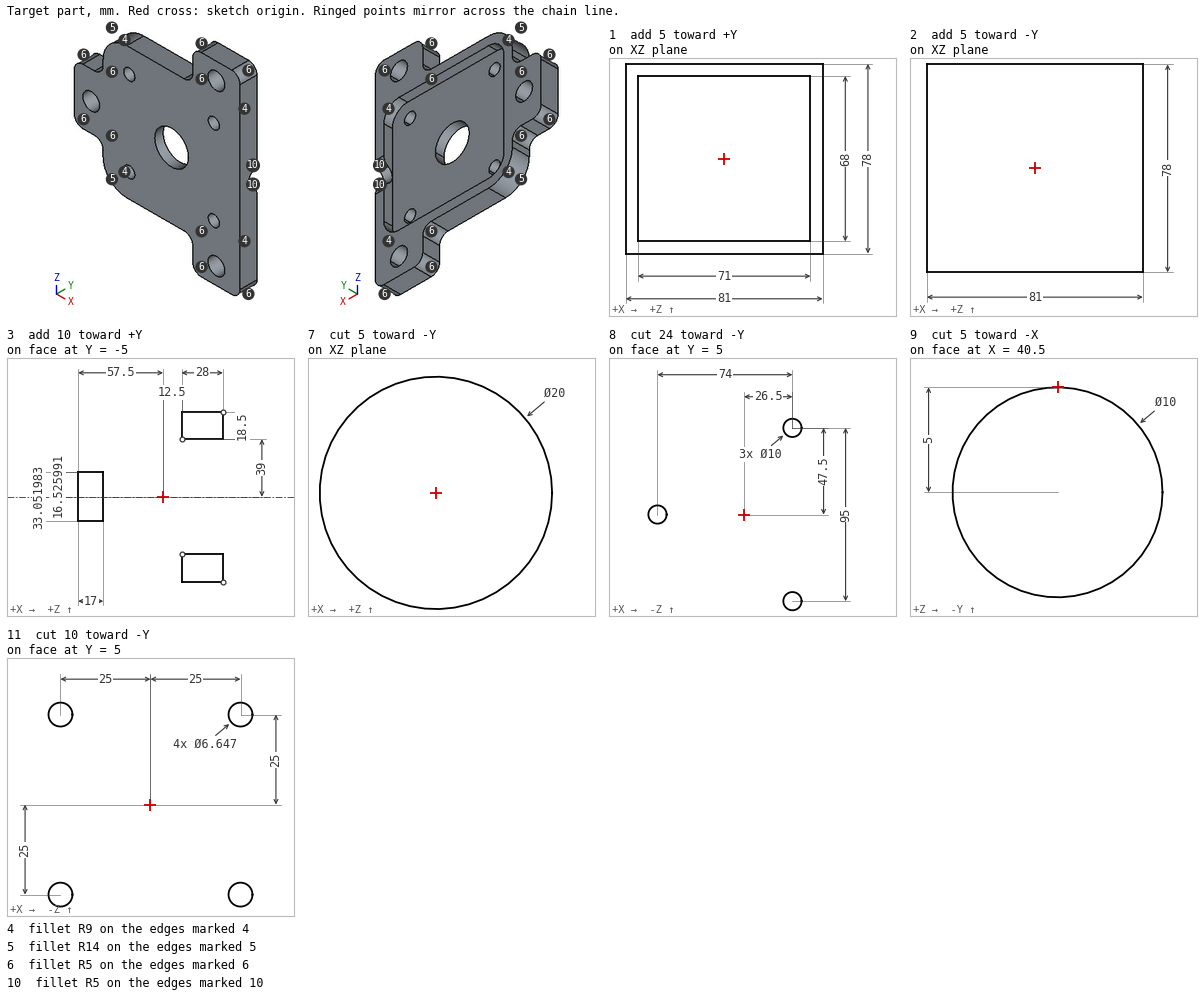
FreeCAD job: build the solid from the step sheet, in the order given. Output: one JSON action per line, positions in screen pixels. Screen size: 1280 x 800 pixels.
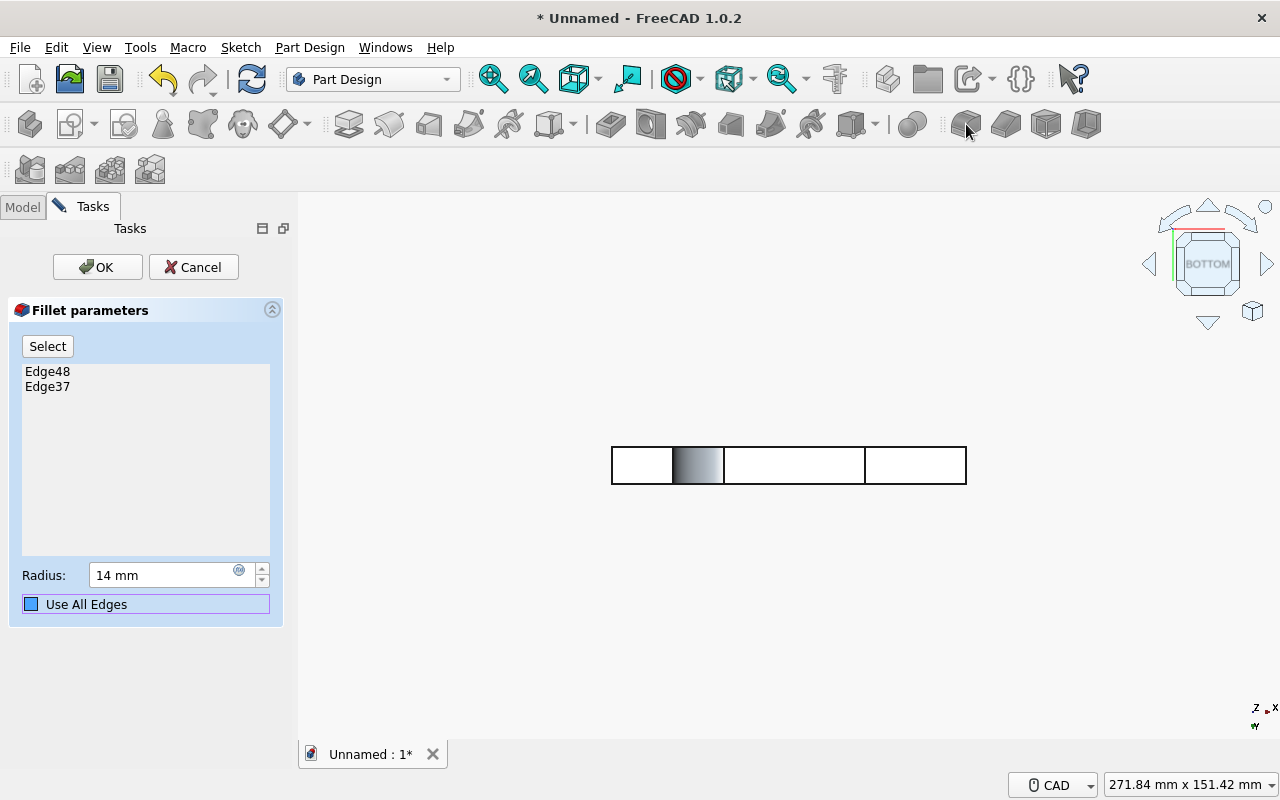
{"action": "left_click", "coordinate": [98, 267]}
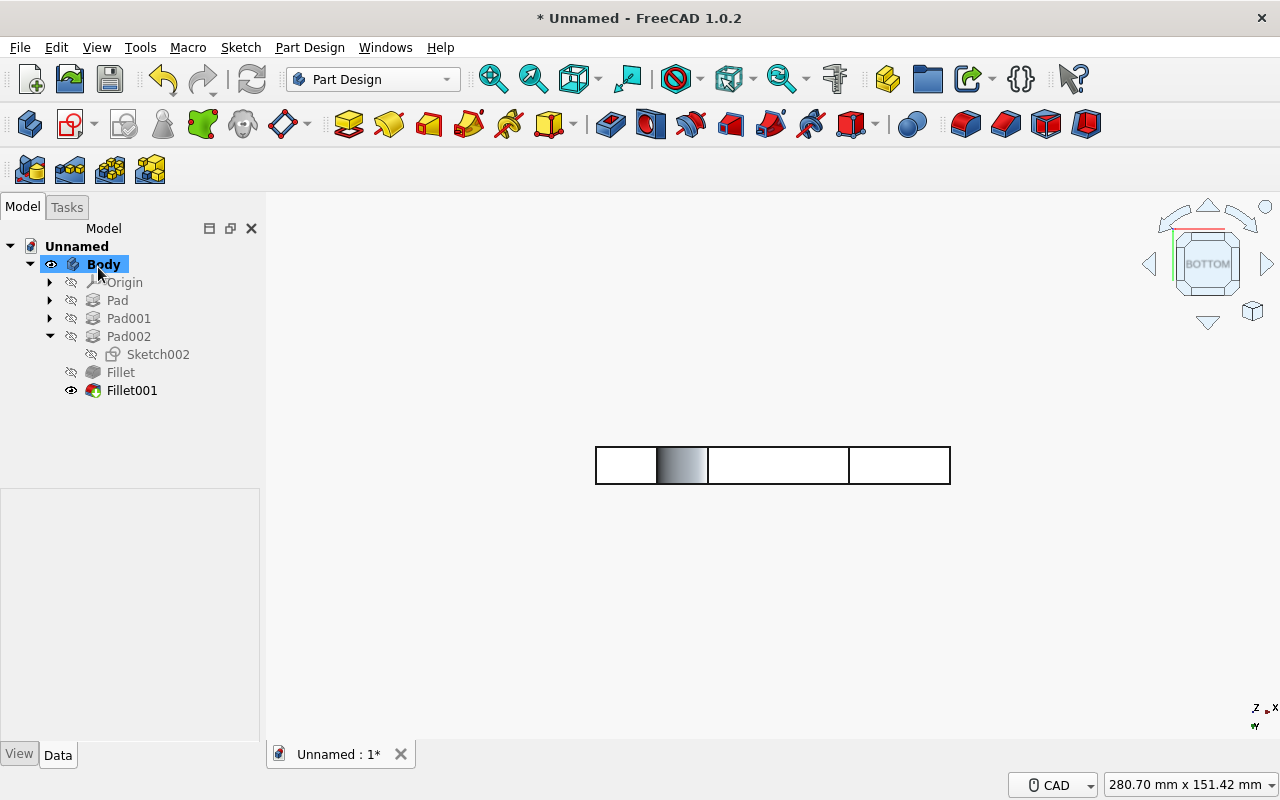
{"action": "left_click", "coordinate": [494, 80]}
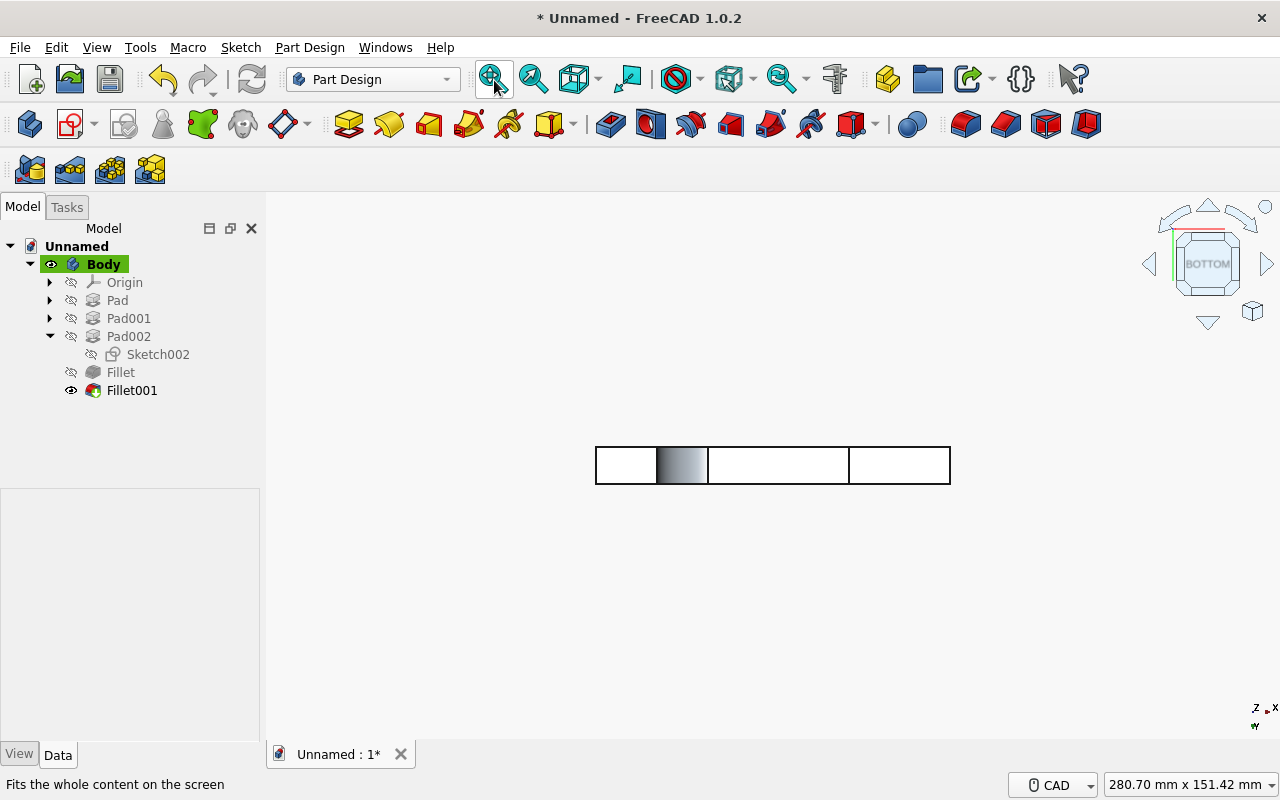
{"action": "left_click", "coordinate": [596, 464]}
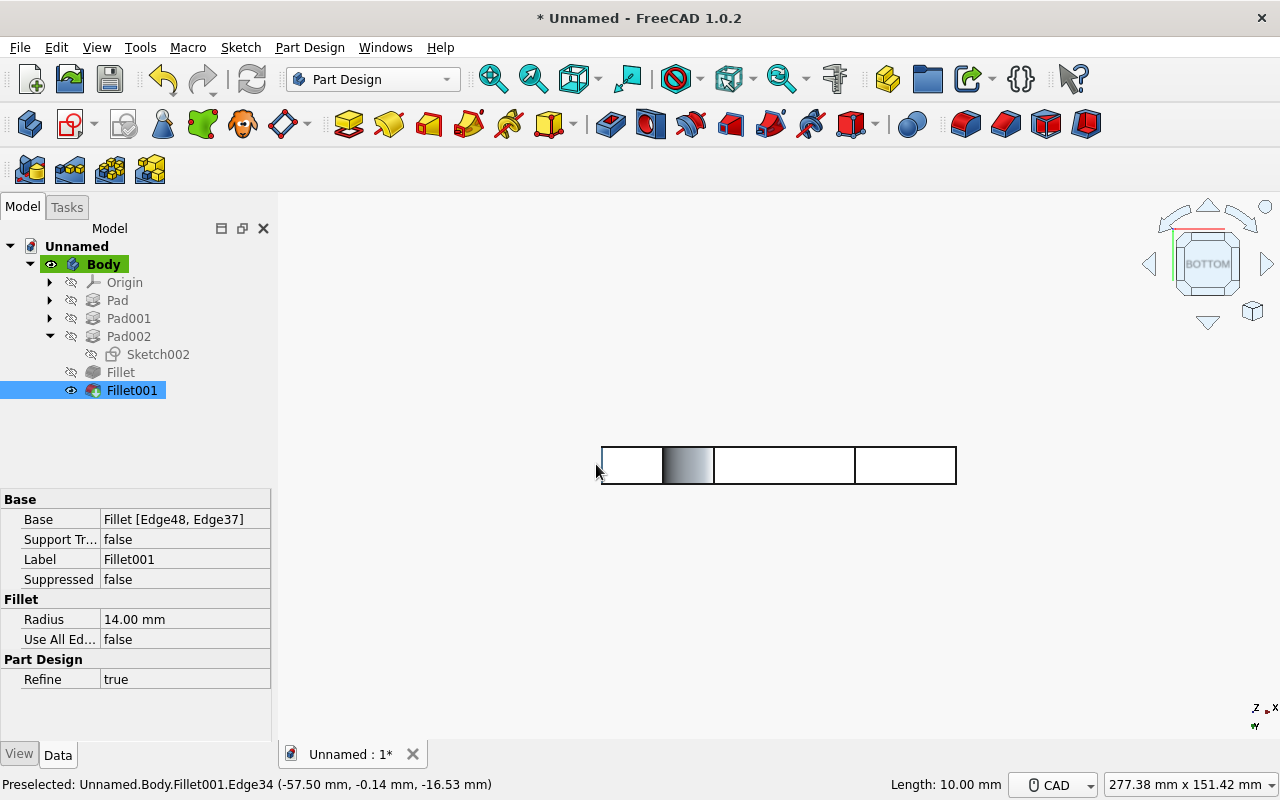
{"action": "left_click", "coordinate": [956, 464], "text": "ctrl"}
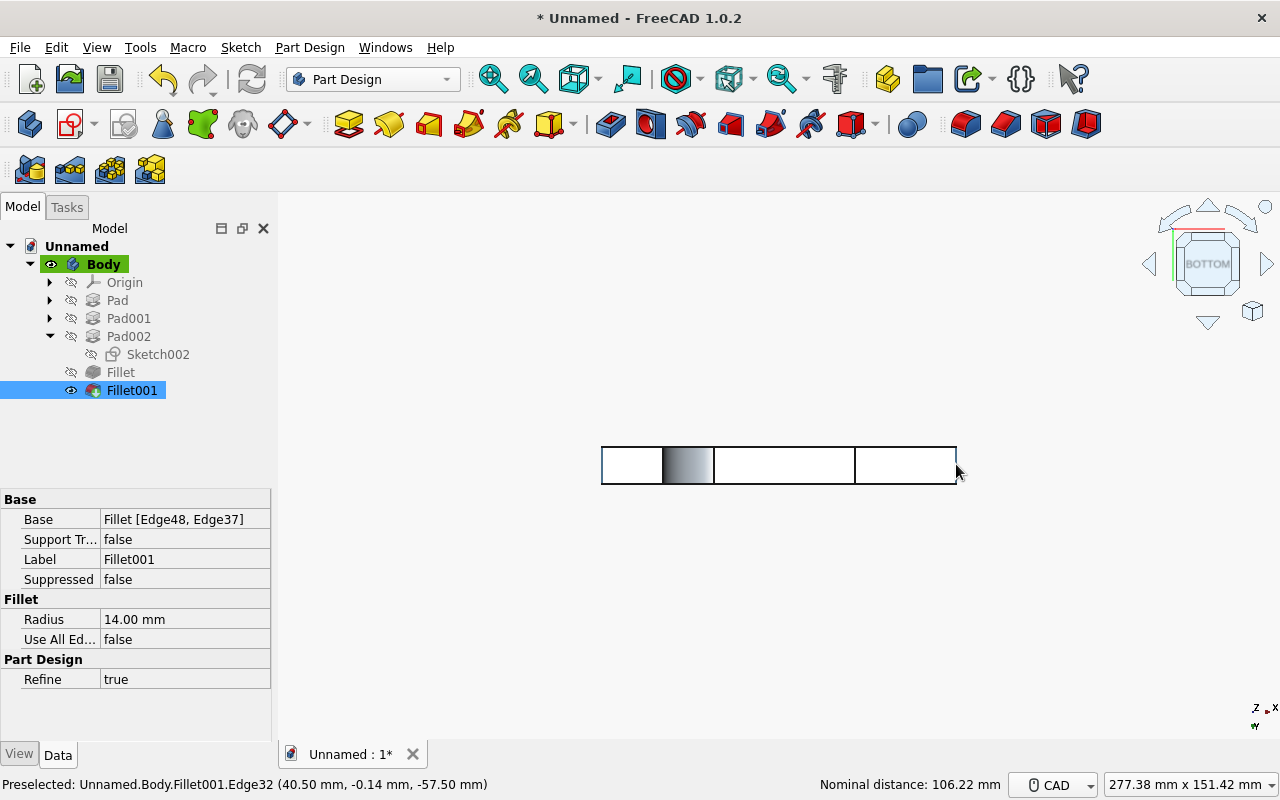
{"action": "left_click", "coordinate": [855, 464], "text": "ctrl"}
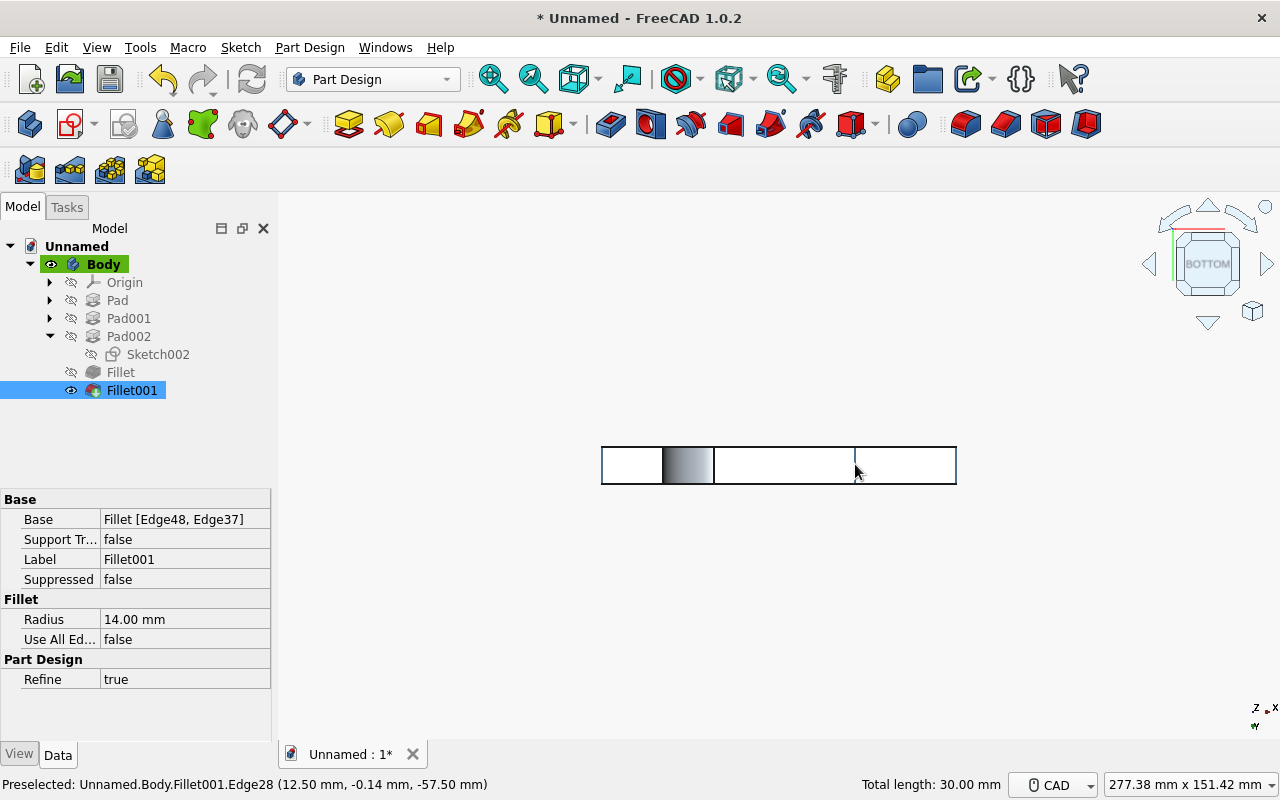
{"action": "key", "text": "0"}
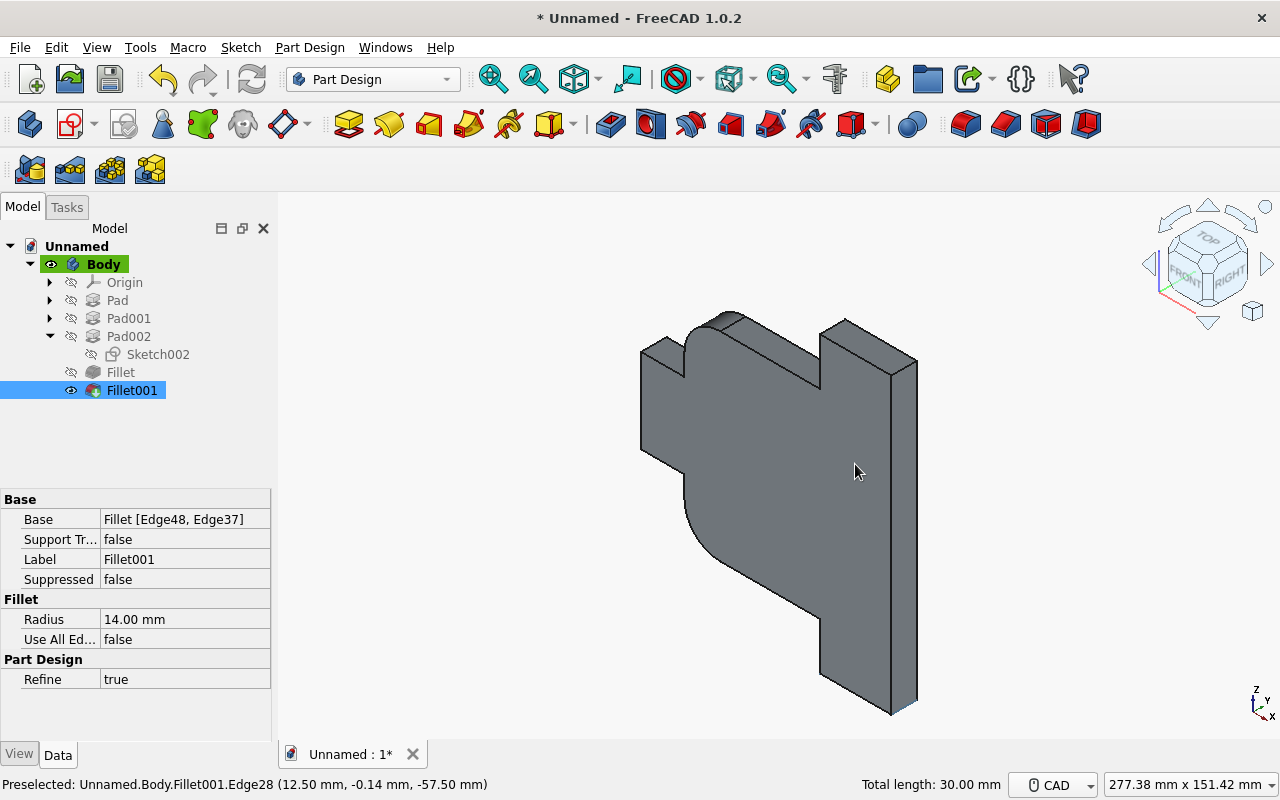
{"action": "left_click", "coordinate": [904, 367], "text": "ctrl"}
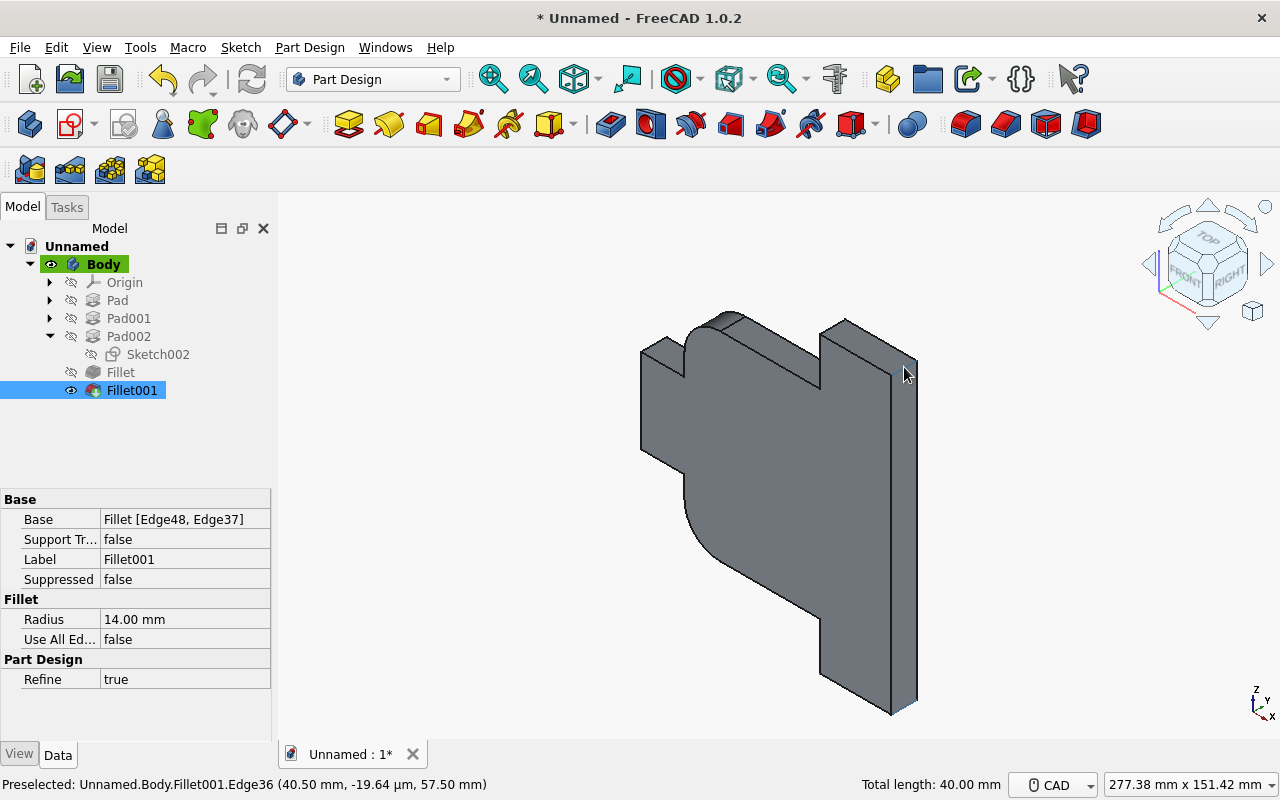
{"action": "key", "text": "2"}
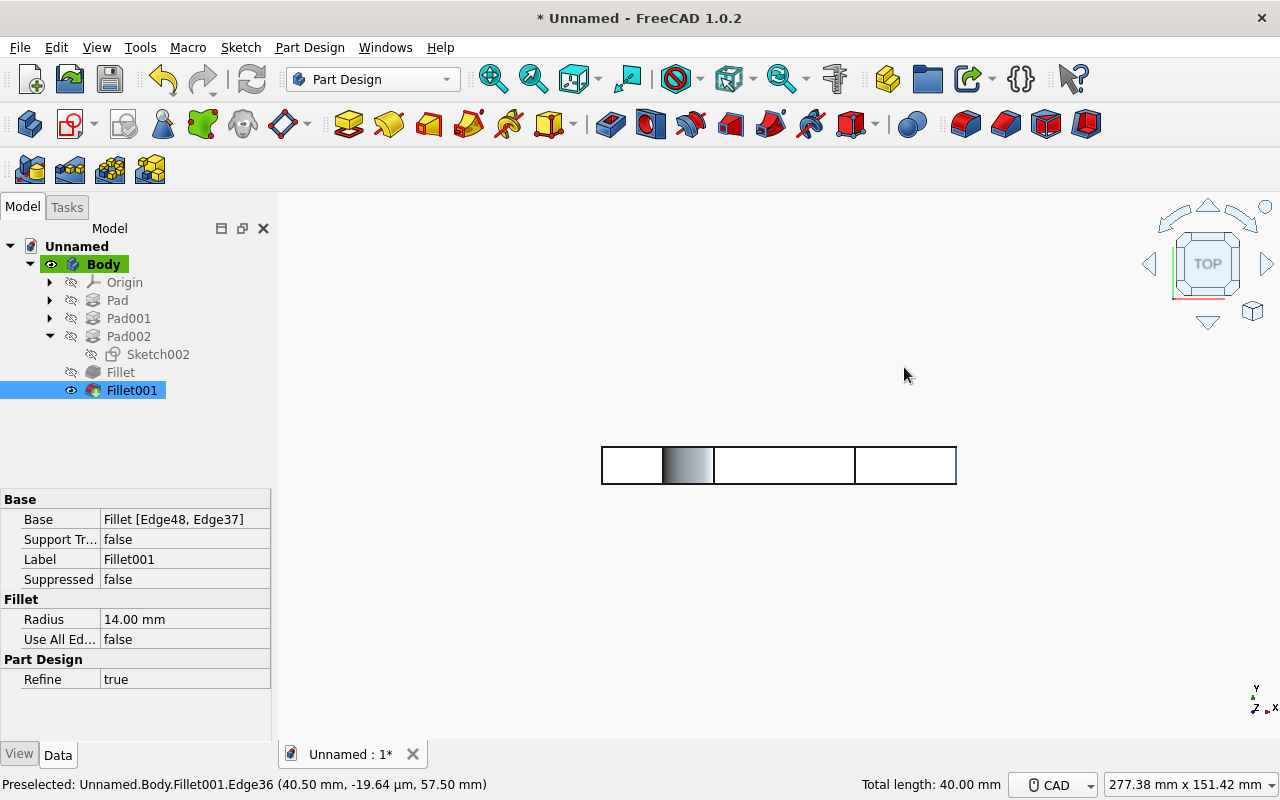
{"action": "key", "text": "v f"}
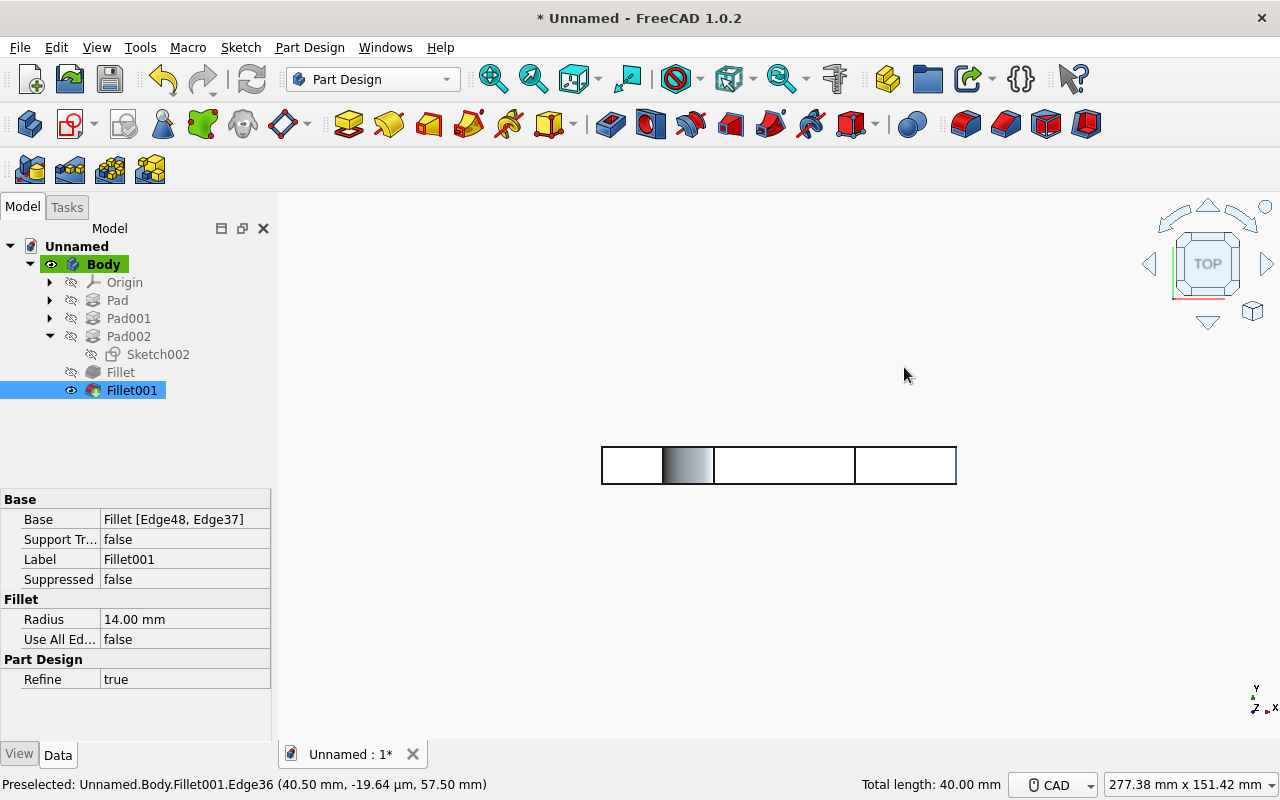
{"action": "left_click", "coordinate": [602, 464], "text": "ctrl"}